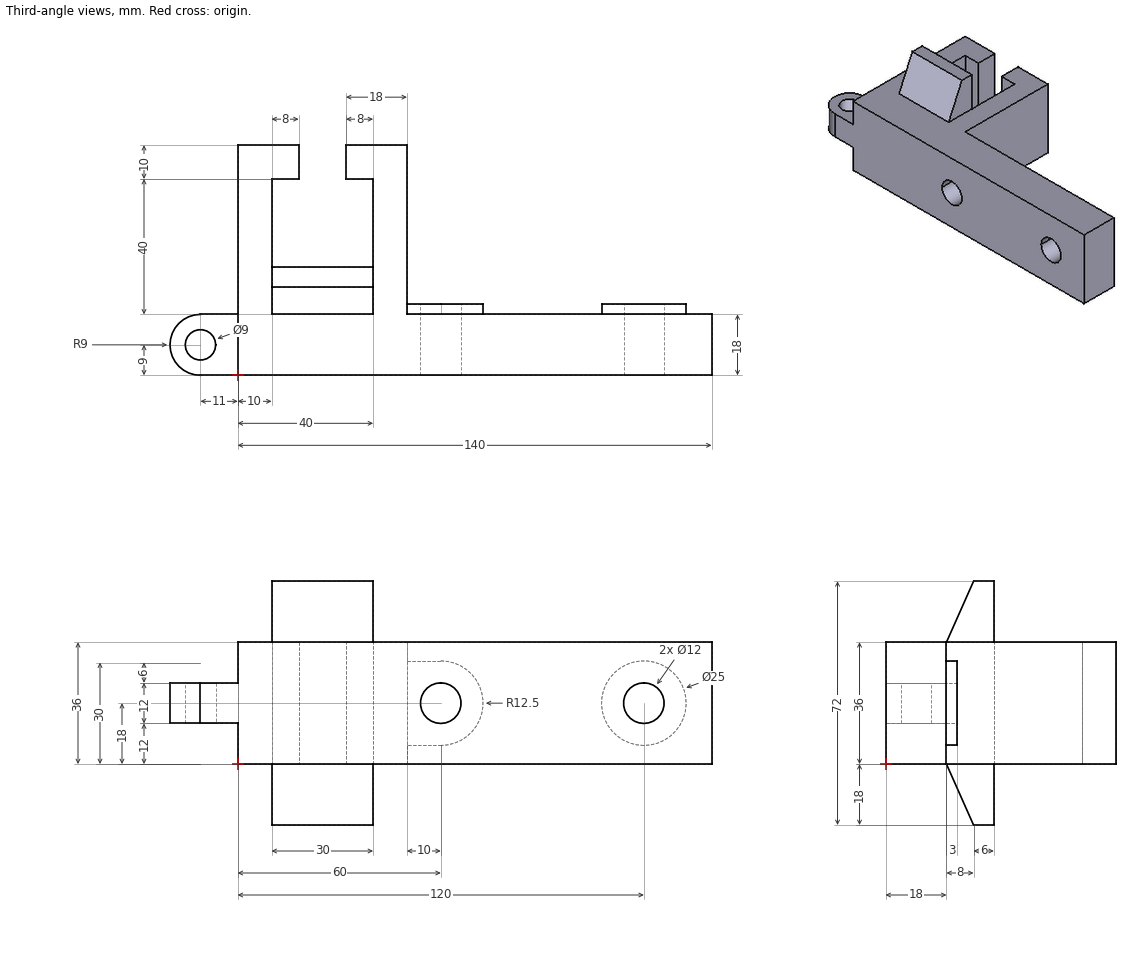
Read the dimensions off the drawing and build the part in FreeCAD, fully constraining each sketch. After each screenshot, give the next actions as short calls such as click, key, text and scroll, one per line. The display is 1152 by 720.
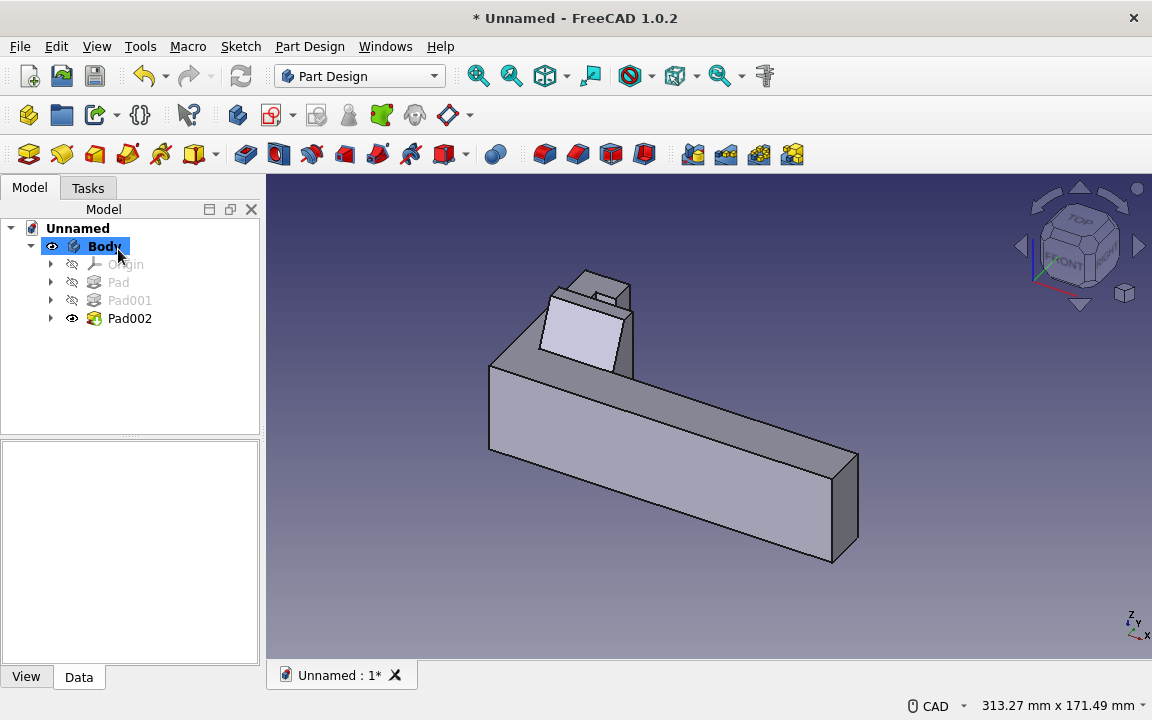
click(270, 116)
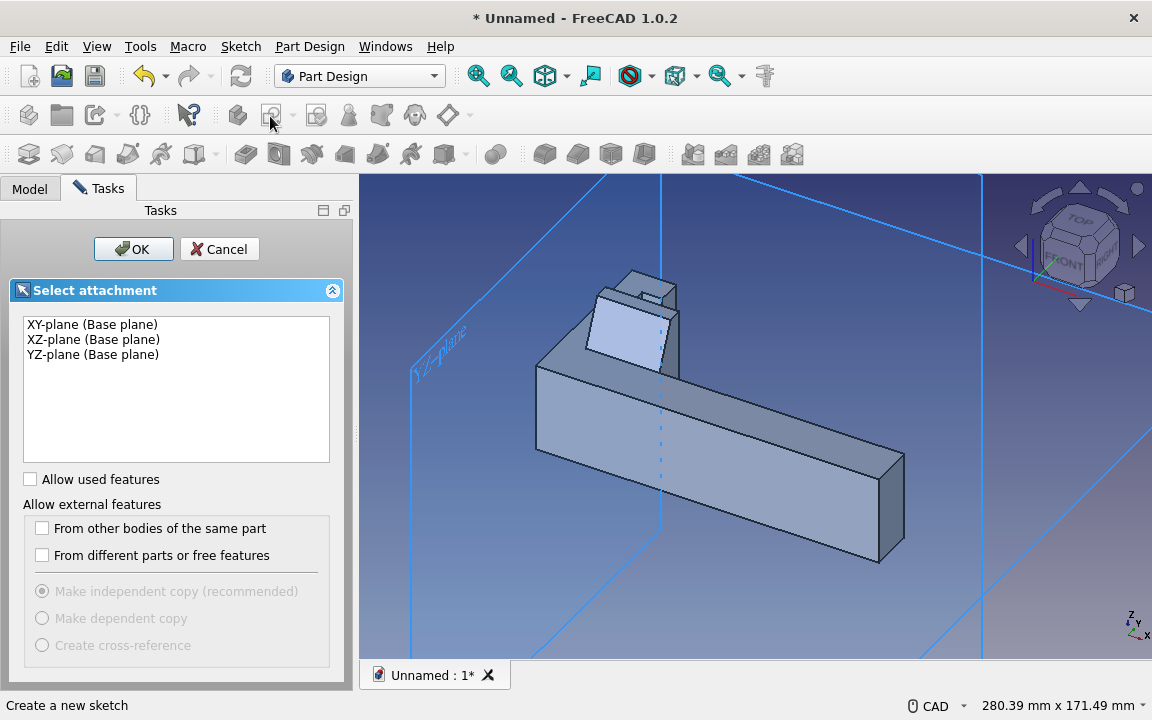
click(84, 324)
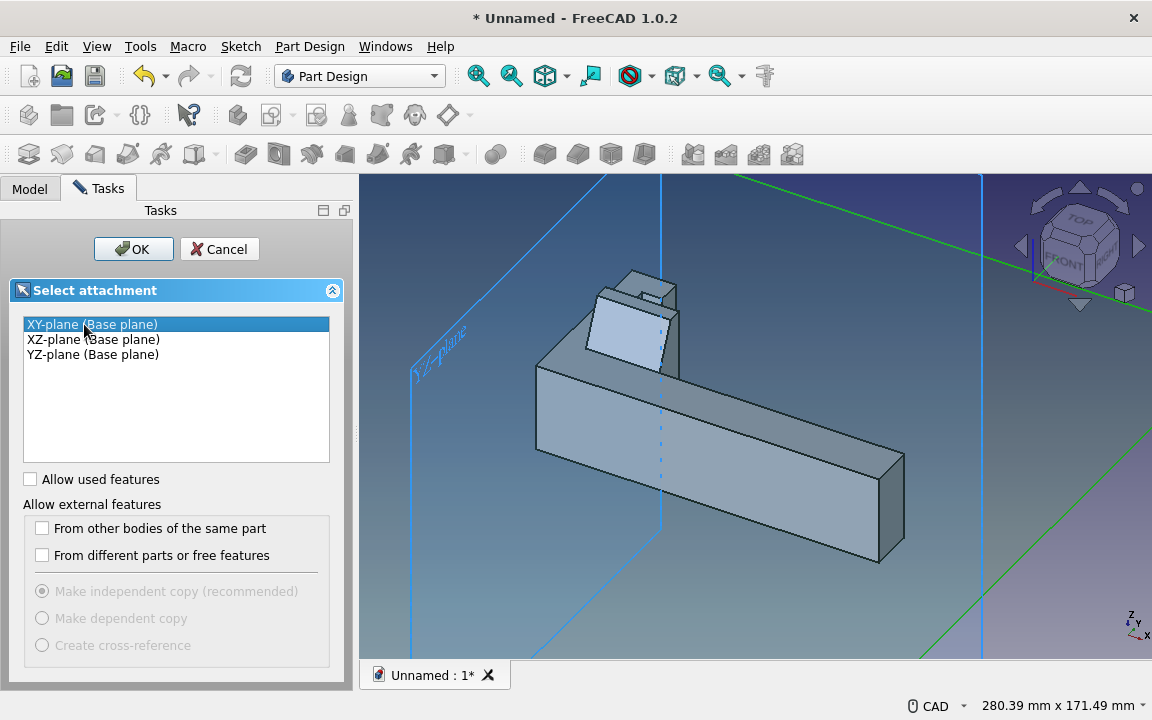
click(134, 249)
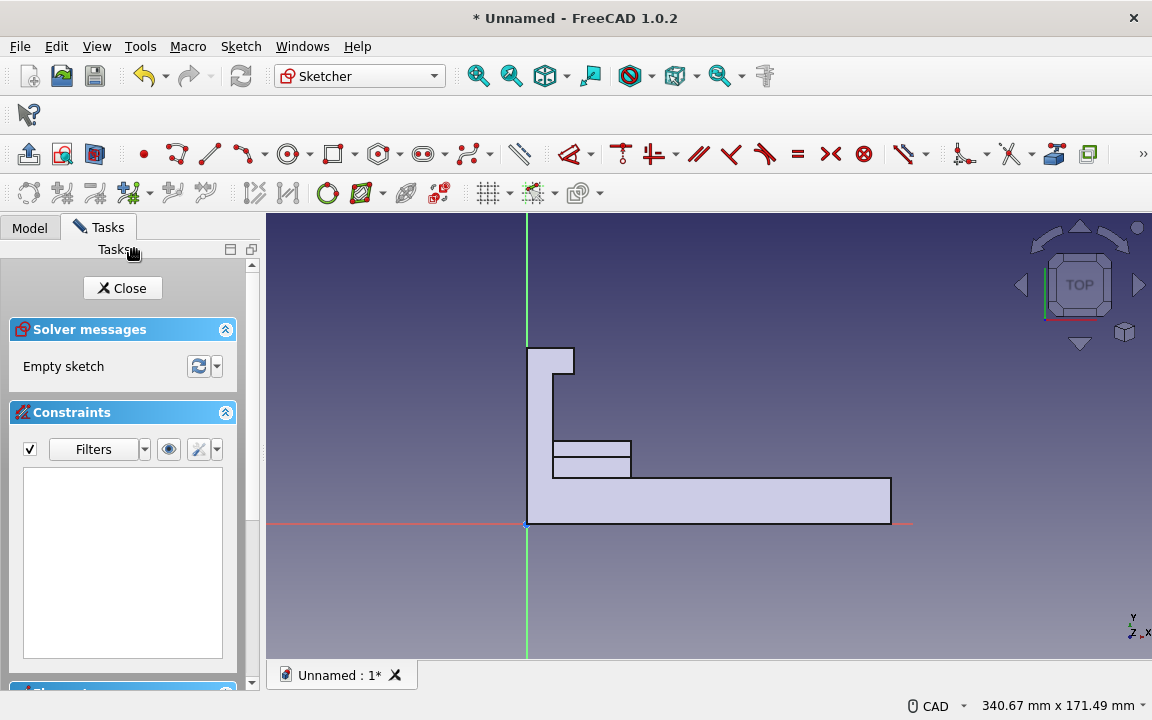
click(95, 154)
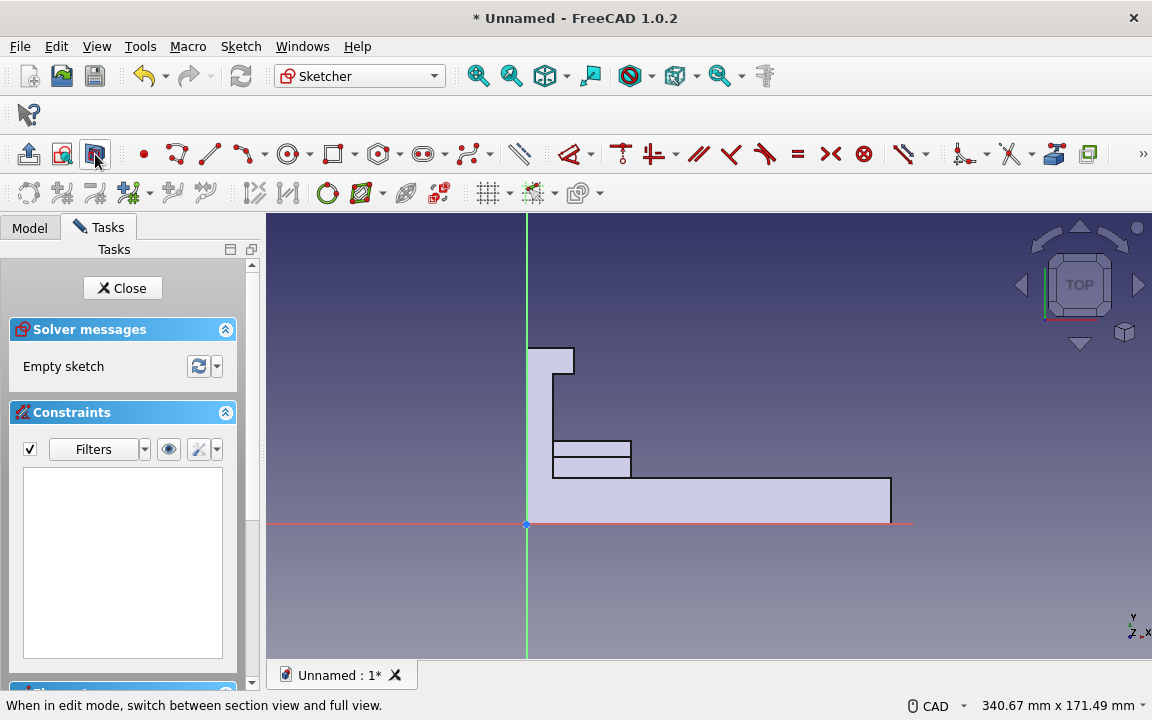
scroll(493, 436, up, 2)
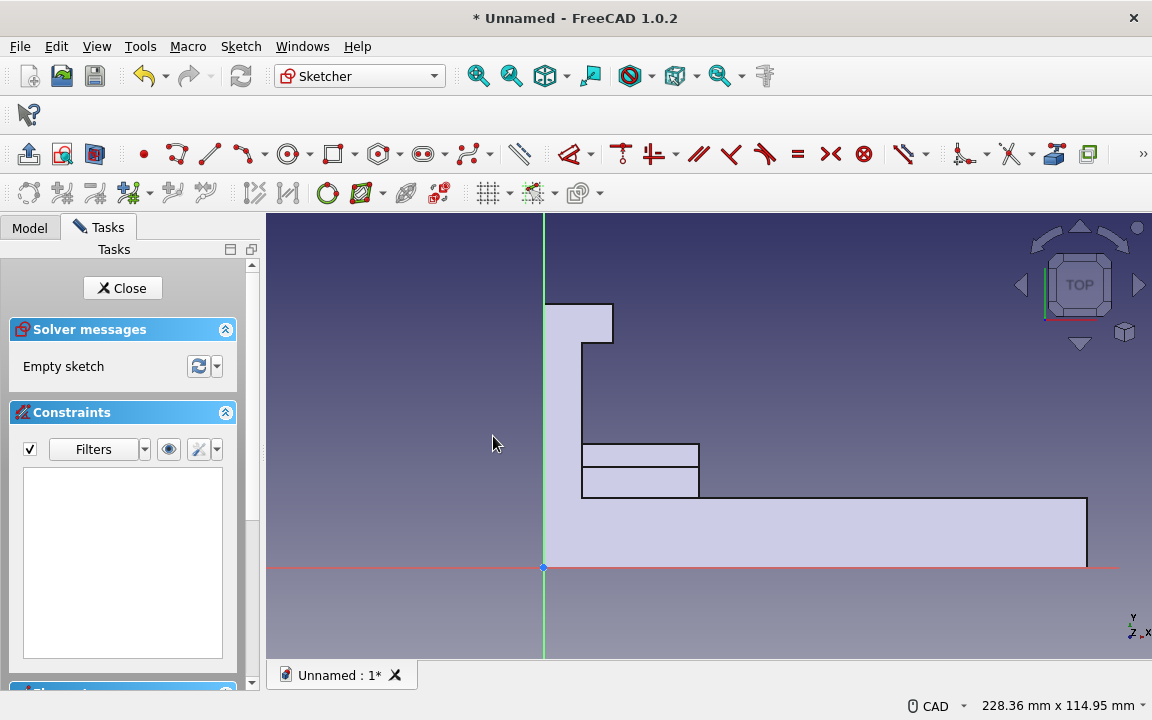
click(177, 154)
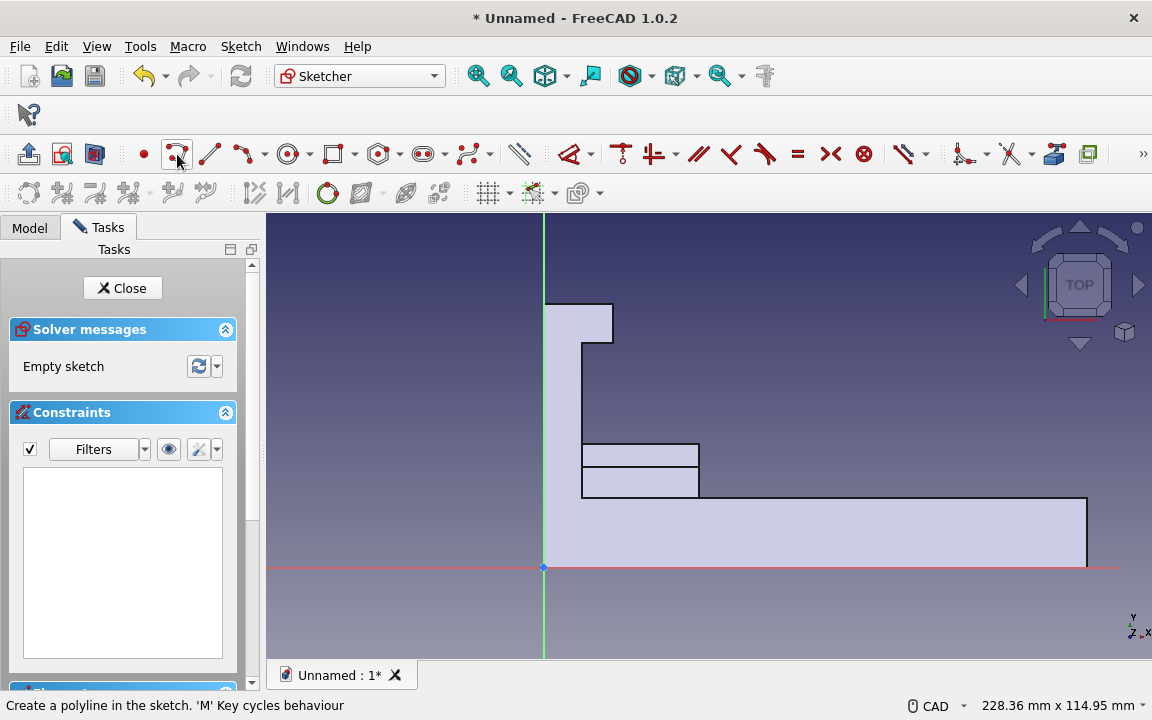
click(699, 498)
click(699, 343)
click(668, 343)
click(668, 304)
click(738, 304)
click(738, 498)
click(699, 499)
key(Escape)
key(Escape)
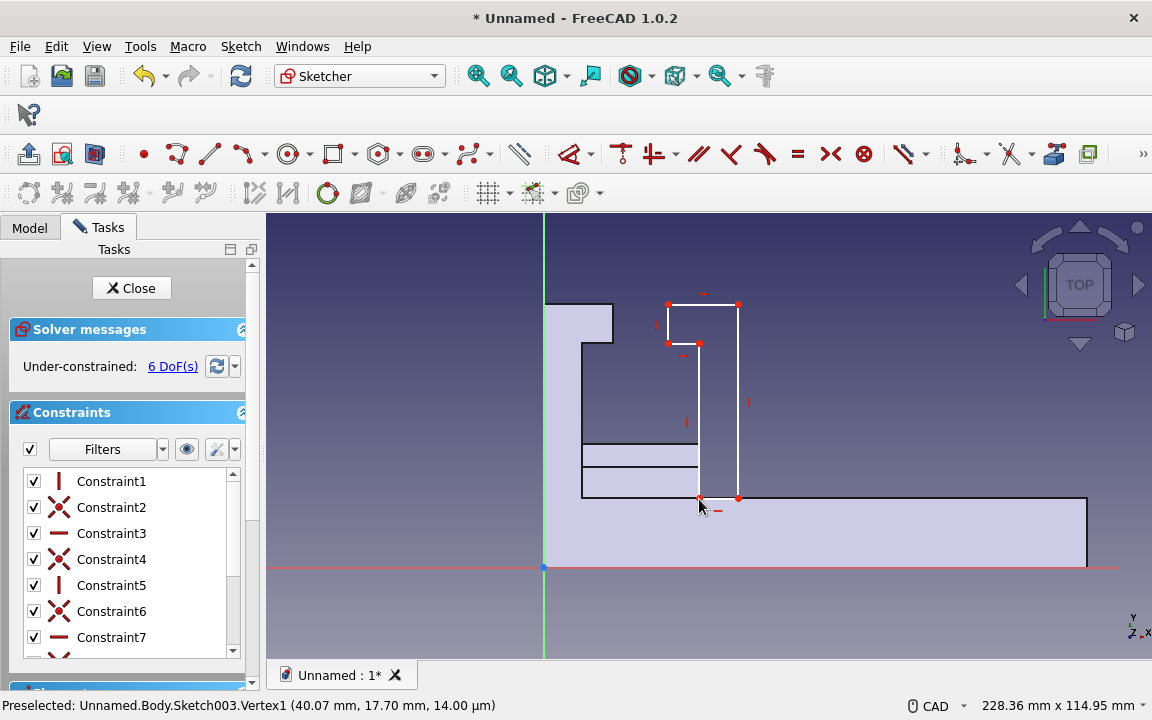
click(568, 154)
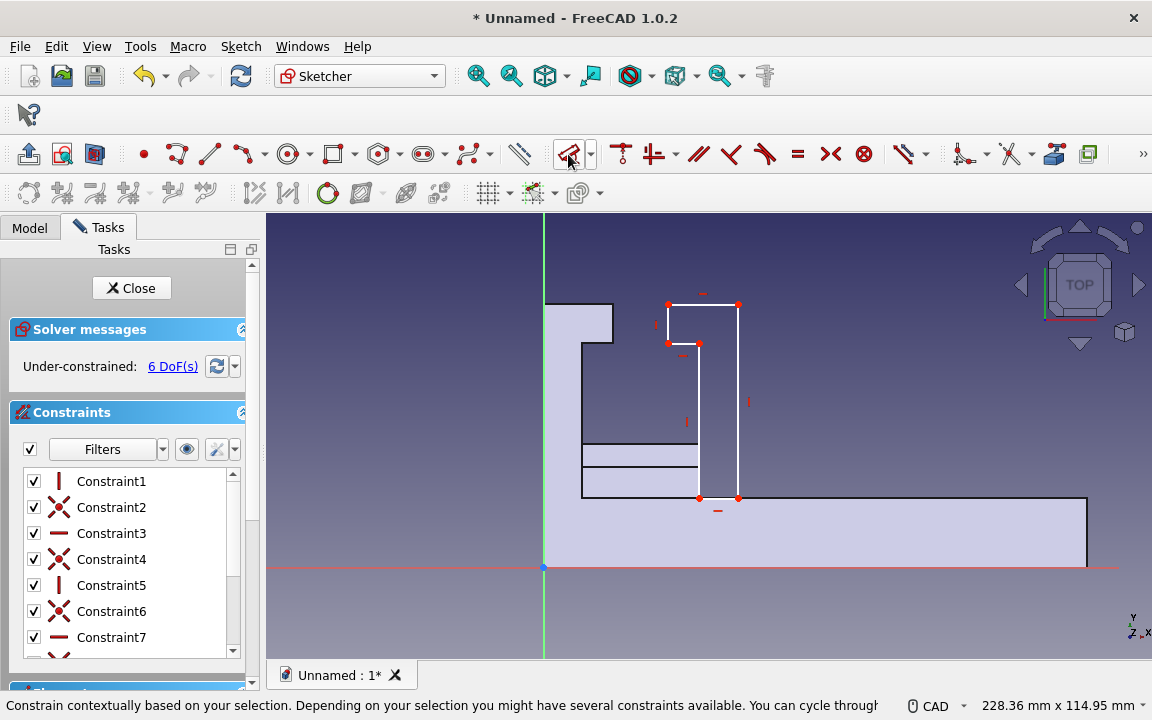
scroll(690, 344, up, 2)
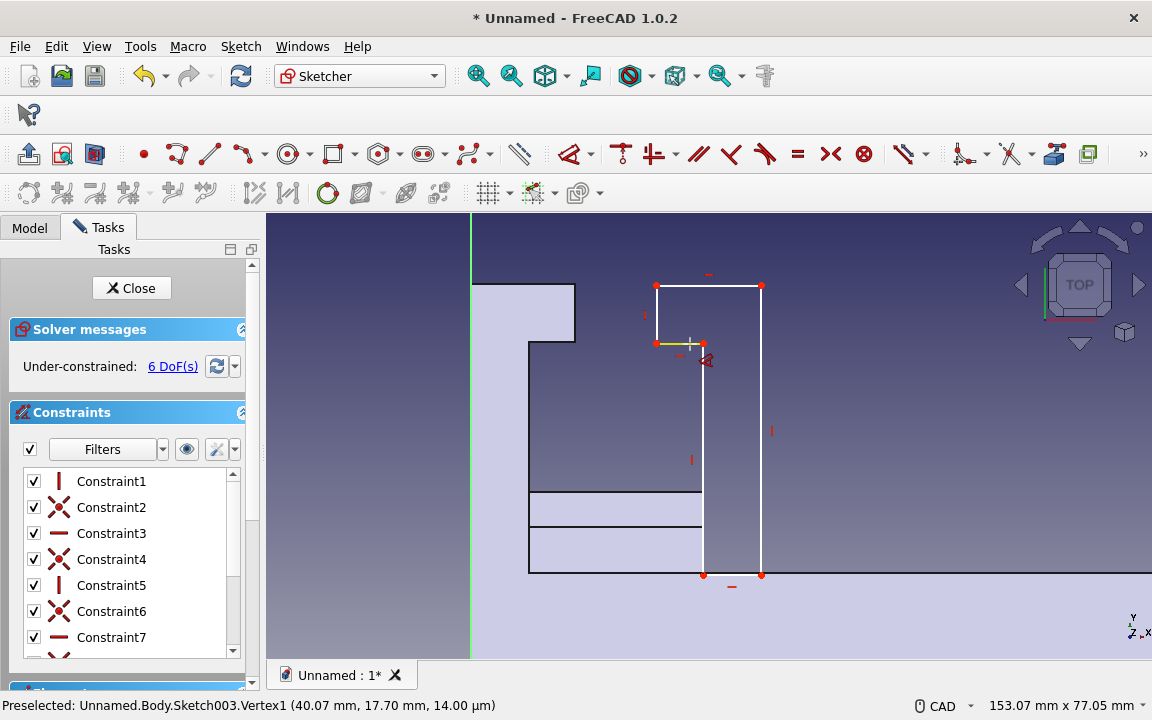
click(689, 344)
click(680, 310)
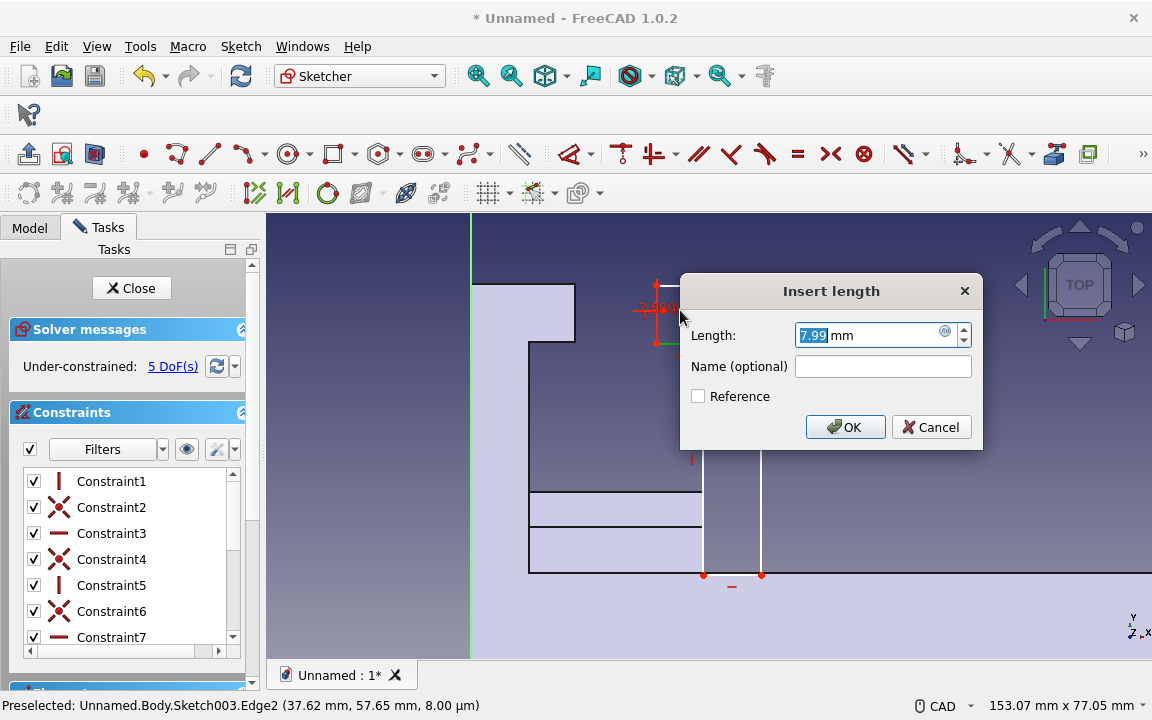
text(8)
key(Return)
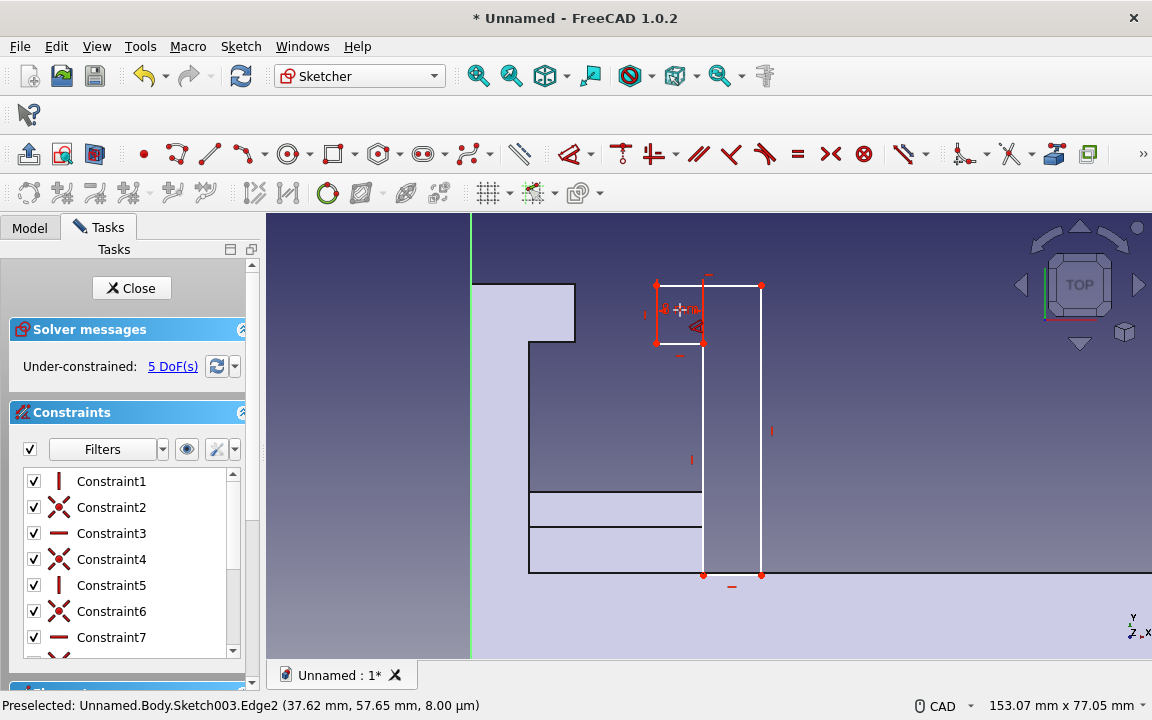
click(703, 506)
click(737, 459)